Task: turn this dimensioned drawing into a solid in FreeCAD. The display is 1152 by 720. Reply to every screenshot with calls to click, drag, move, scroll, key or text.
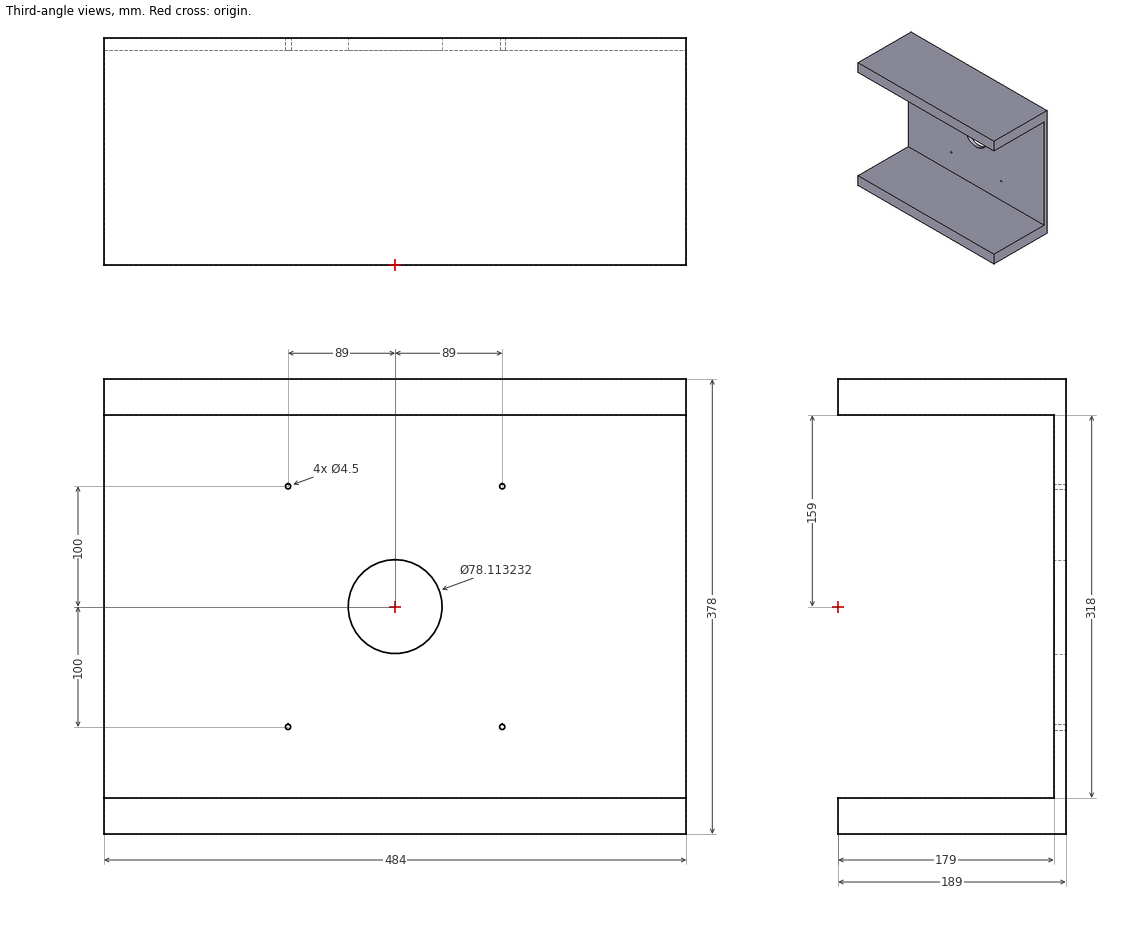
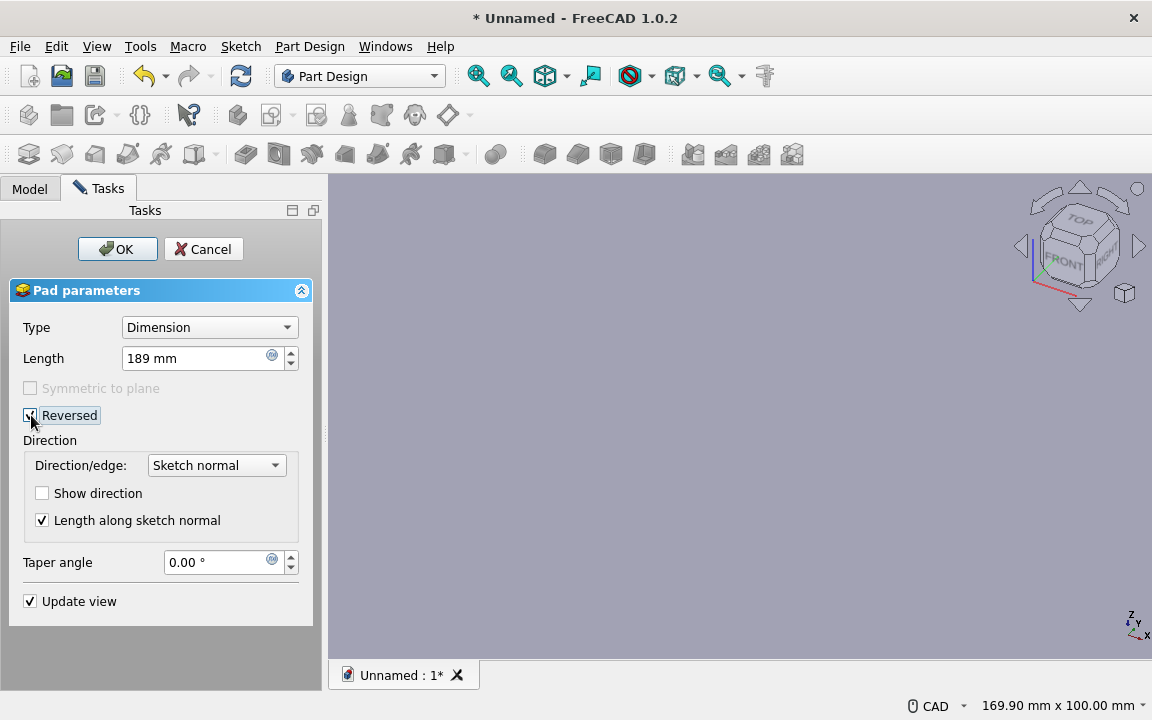
click(118, 249)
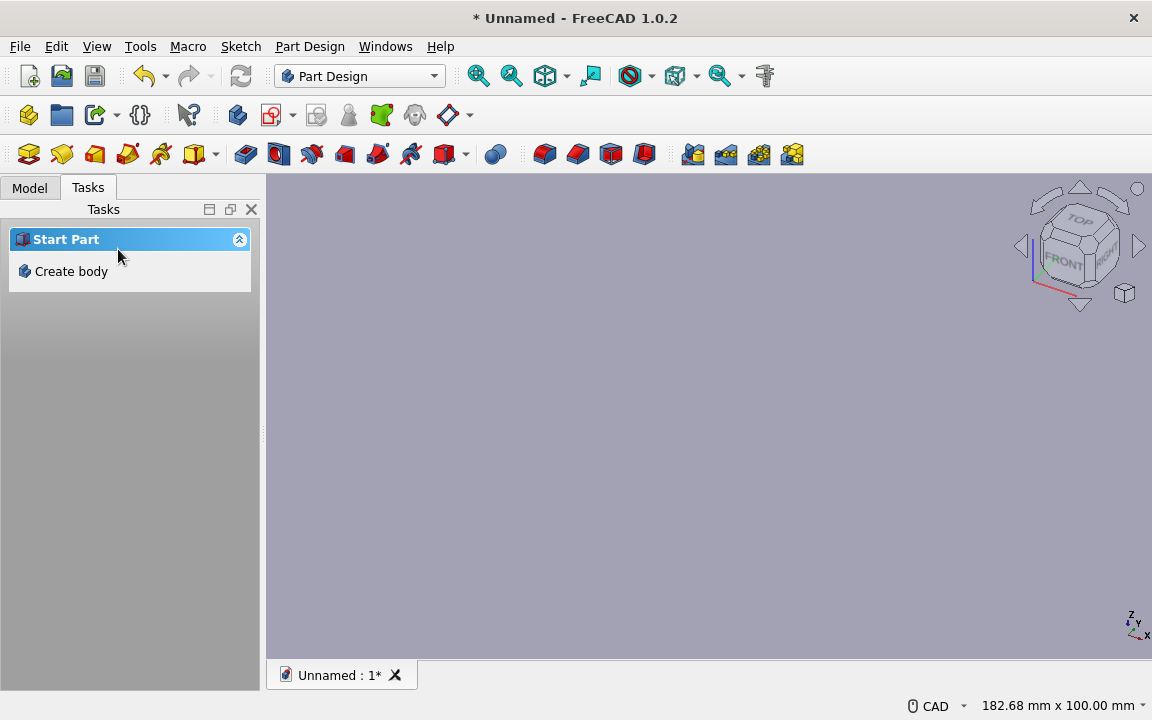
click(479, 76)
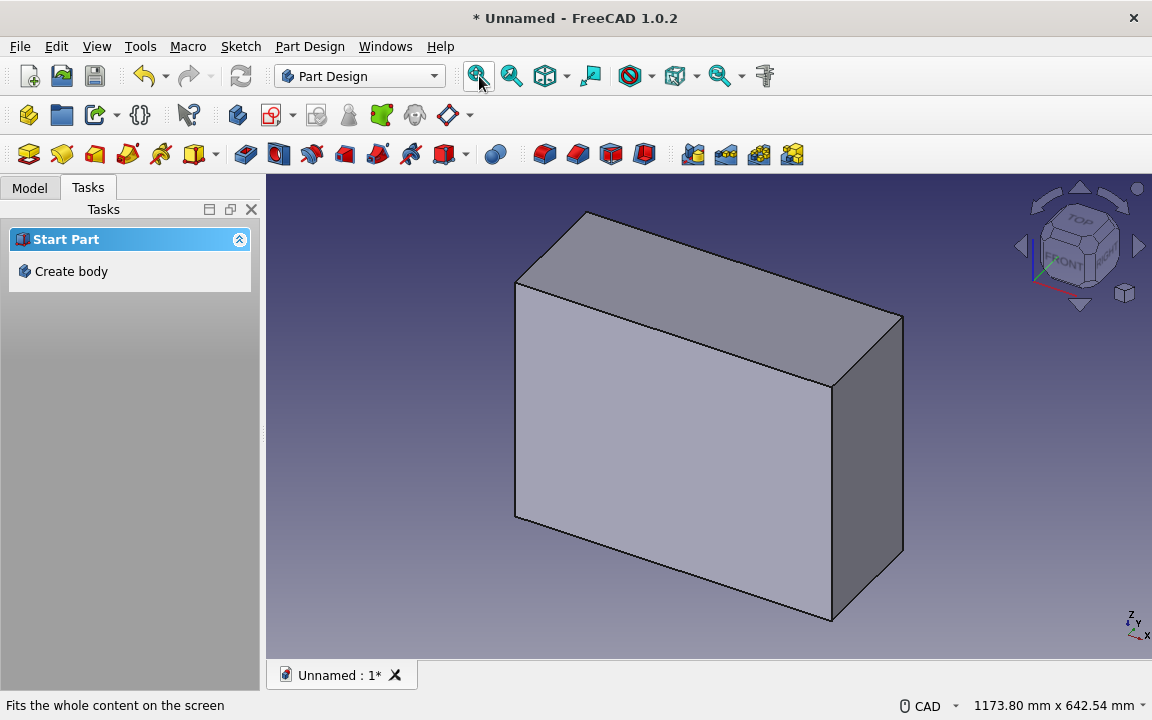
key(6)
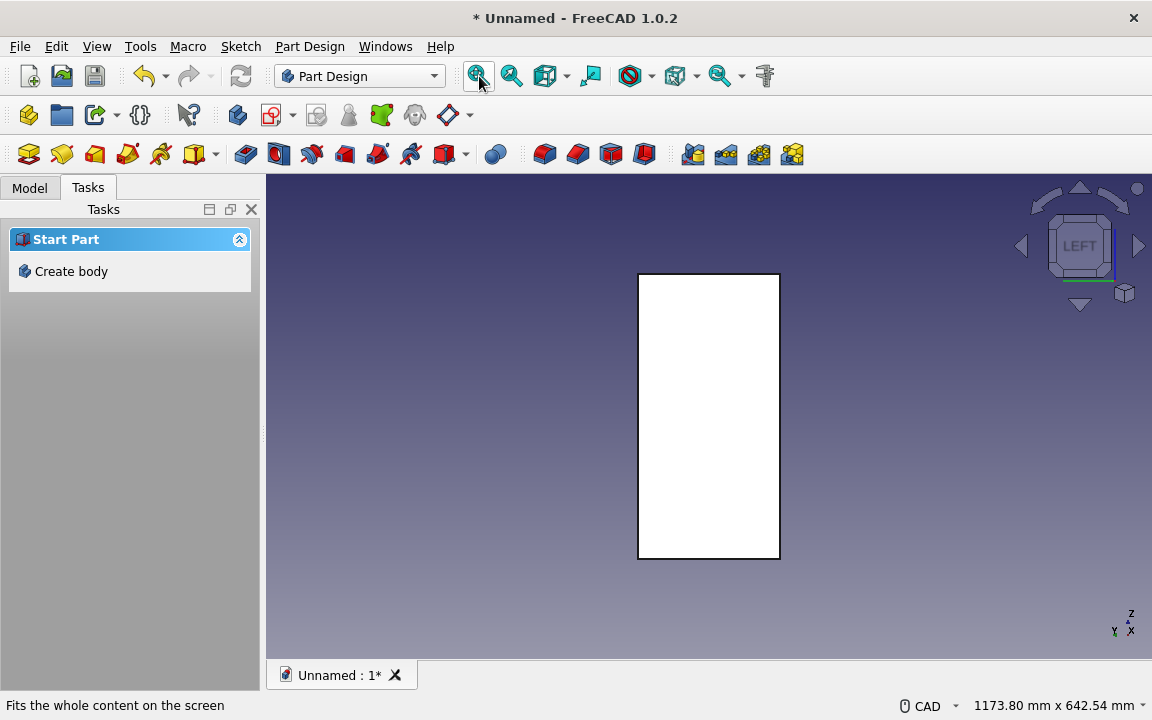
click(709, 415)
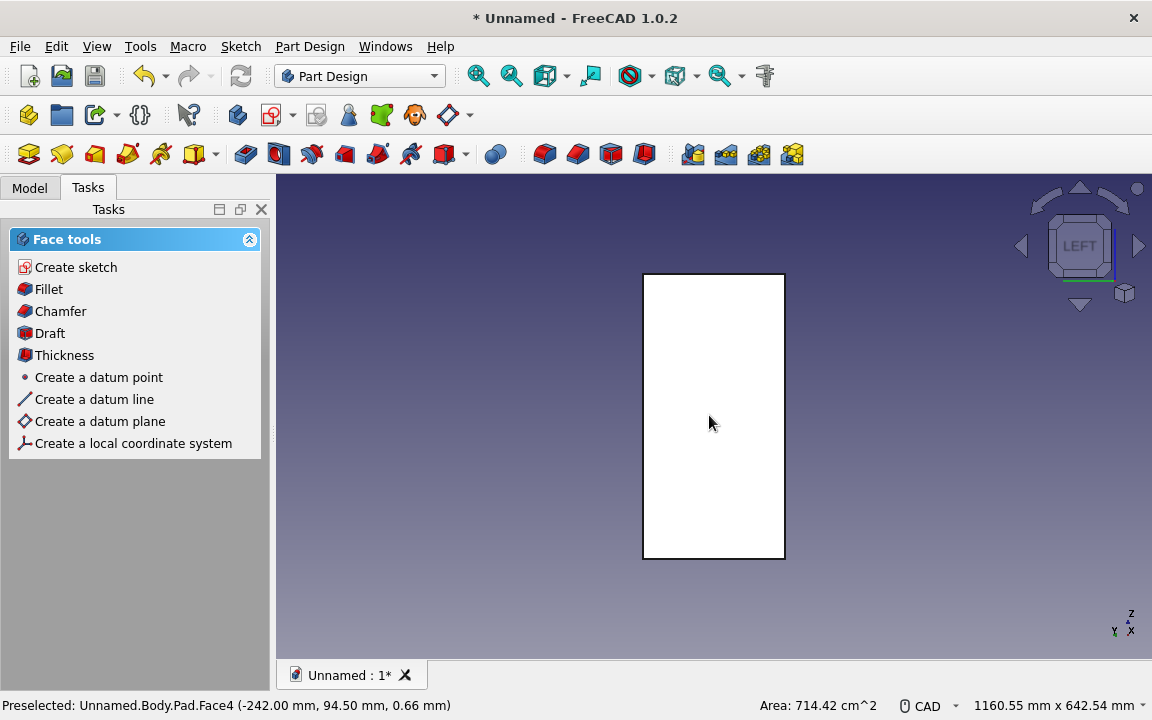
click(270, 116)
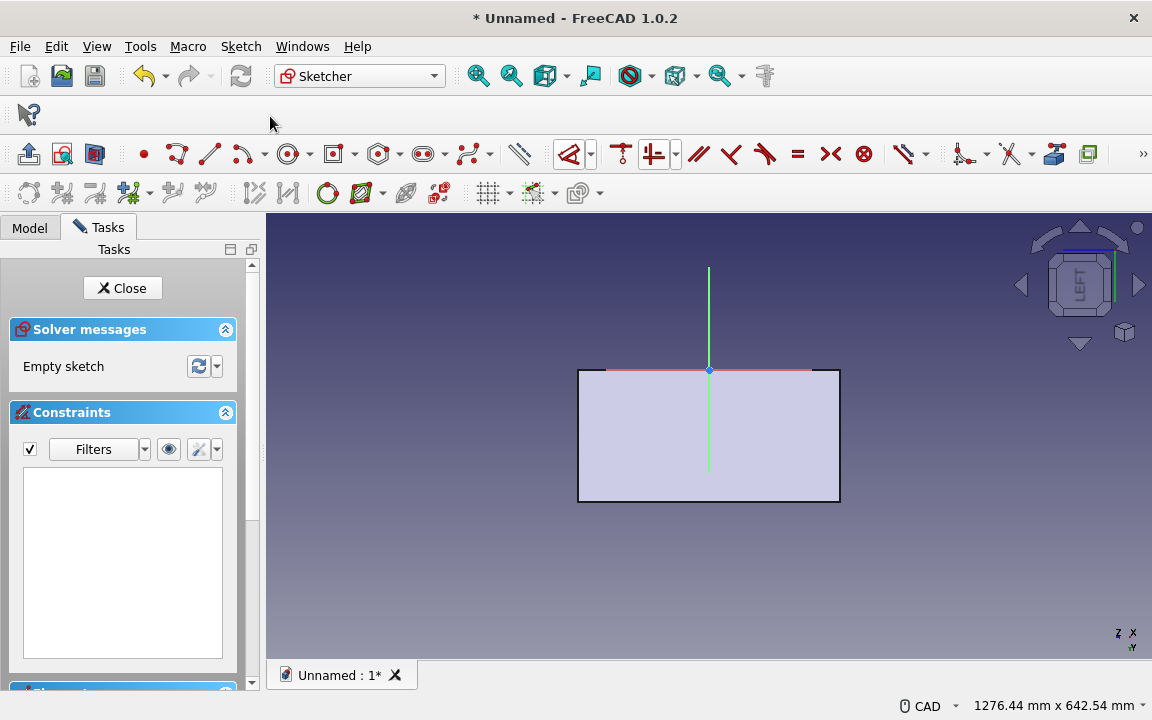
scroll(765, 430, up, 4)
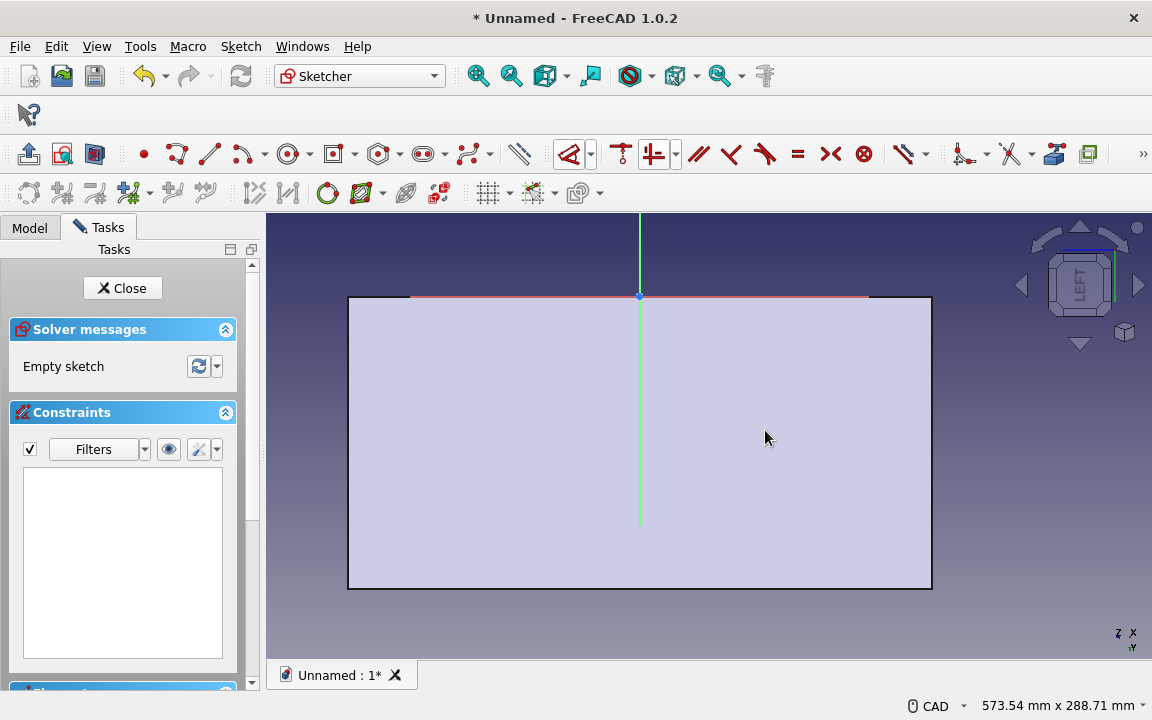
key(g)
key(r)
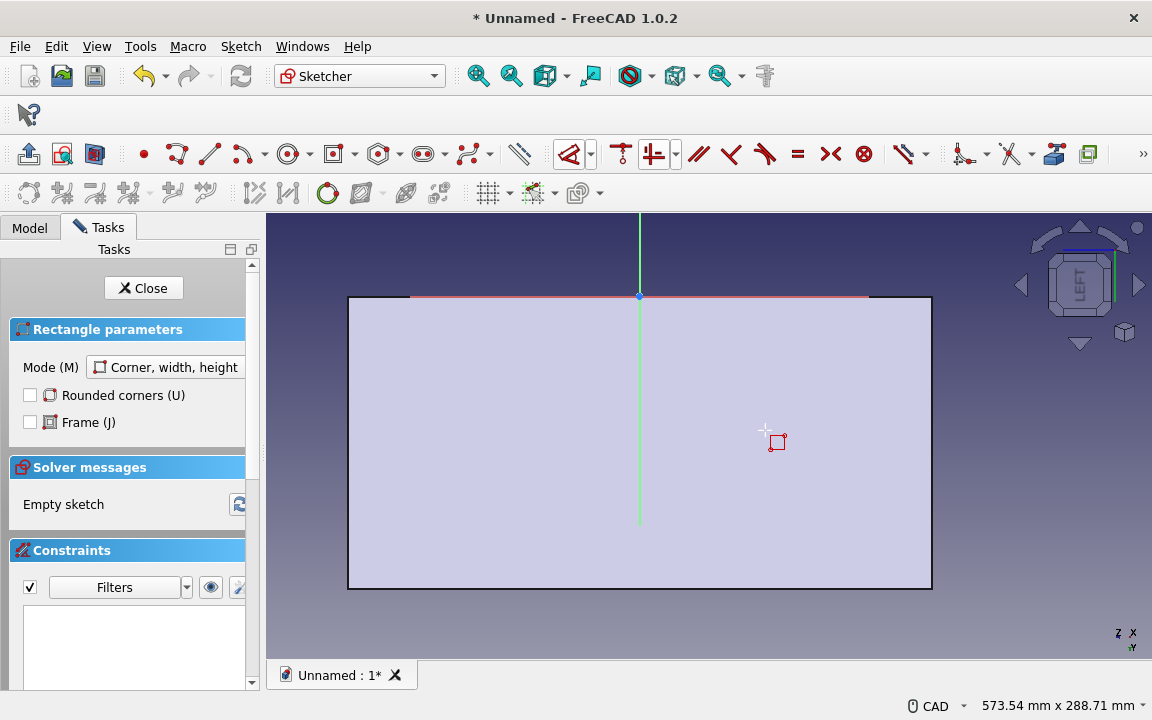
click(394, 297)
move(885, 573)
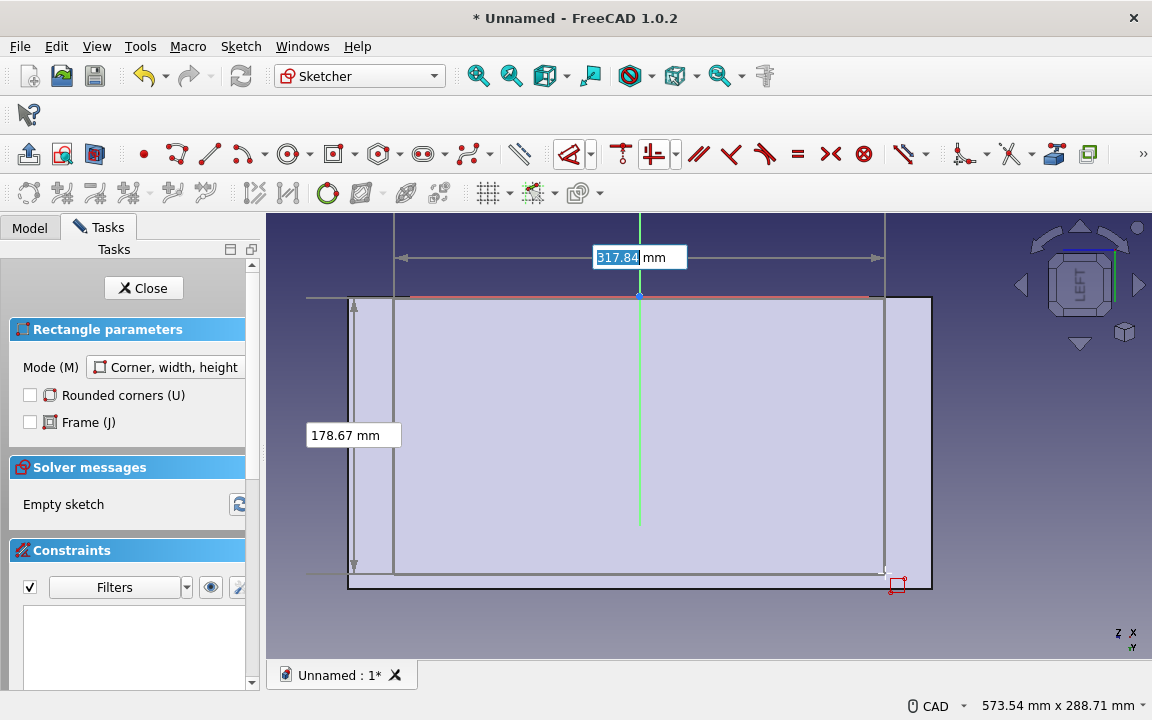
text(318)
key(Tab)
text(179)
key(Return)
key(Escape)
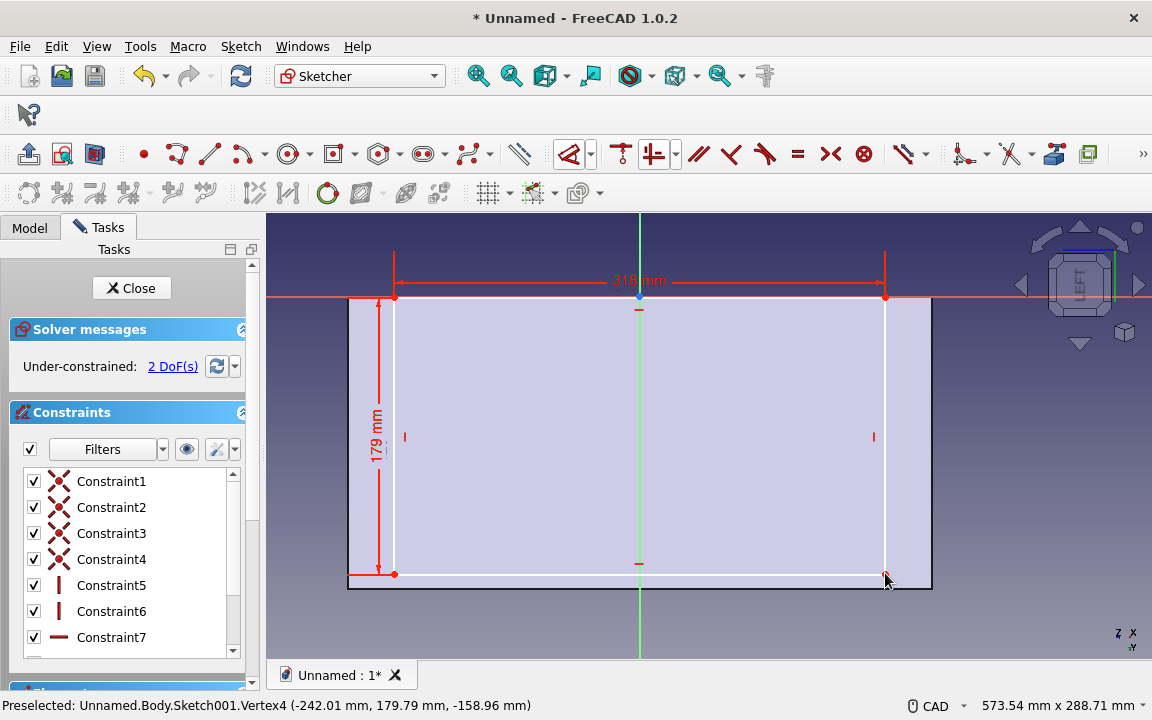
click(394, 298)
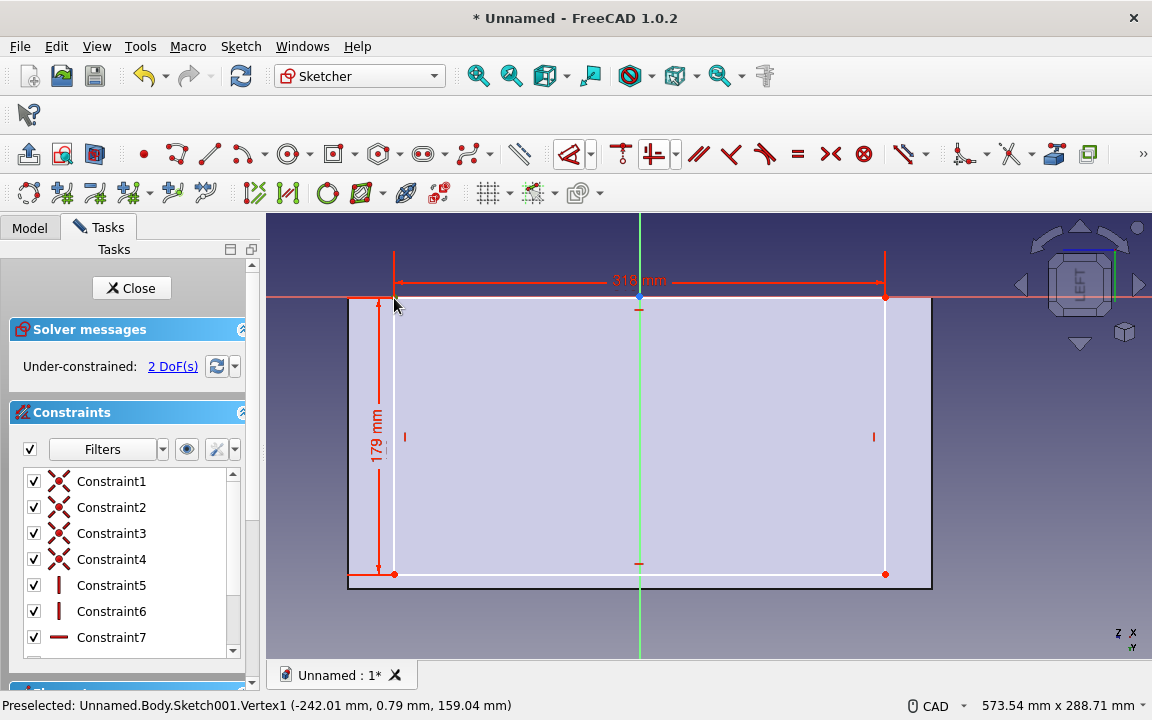
click(344, 297)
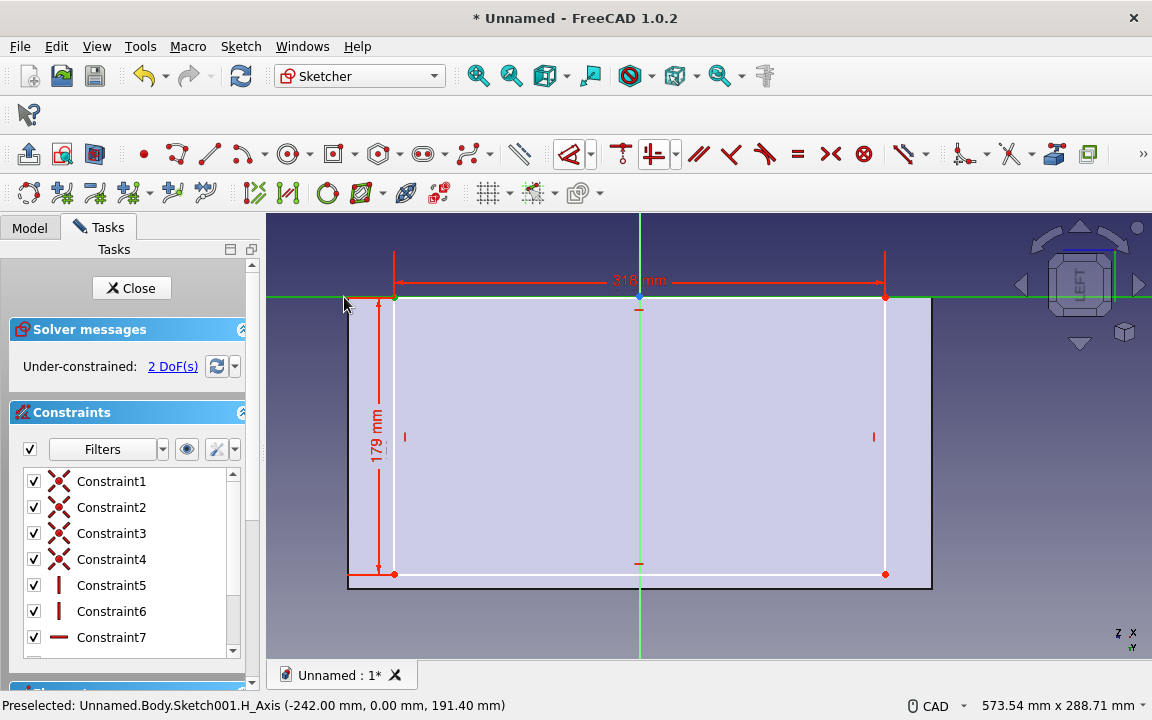
click(621, 154)